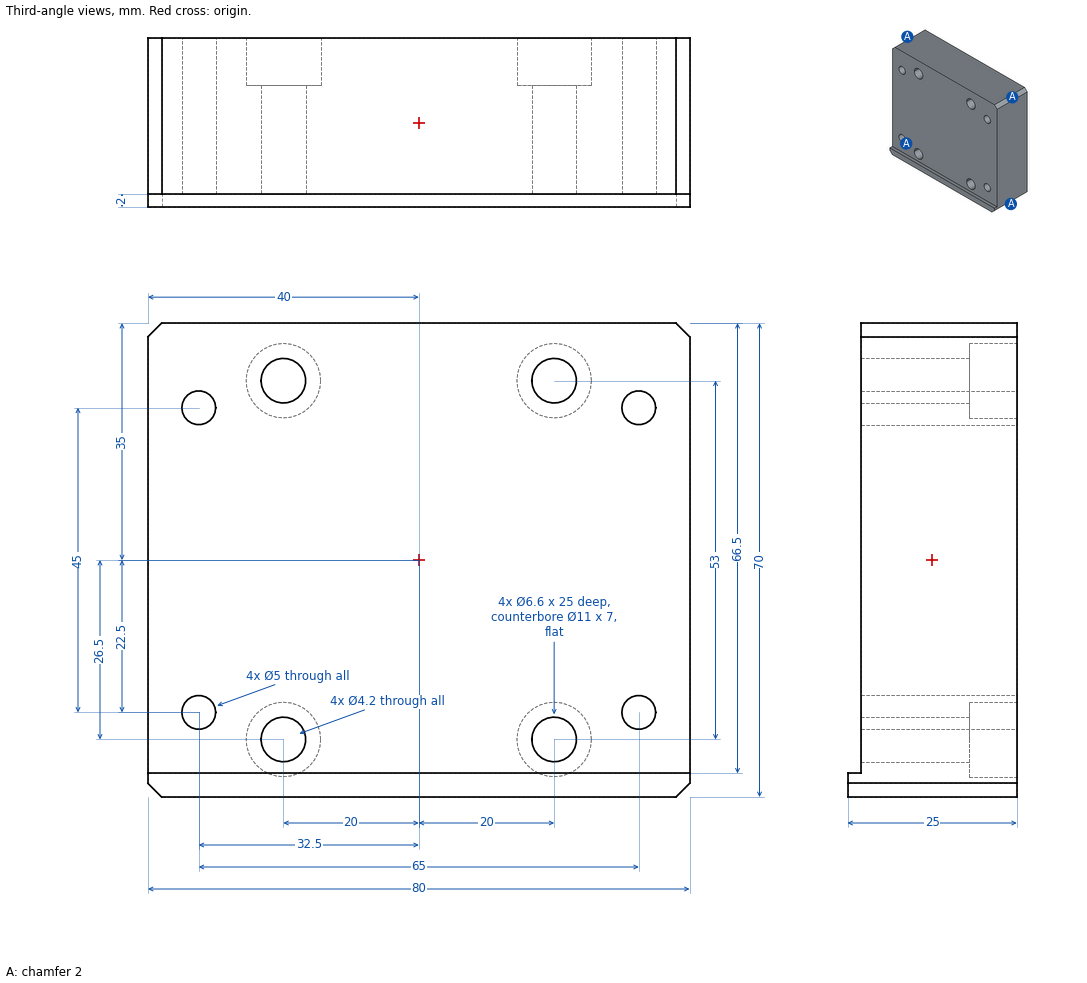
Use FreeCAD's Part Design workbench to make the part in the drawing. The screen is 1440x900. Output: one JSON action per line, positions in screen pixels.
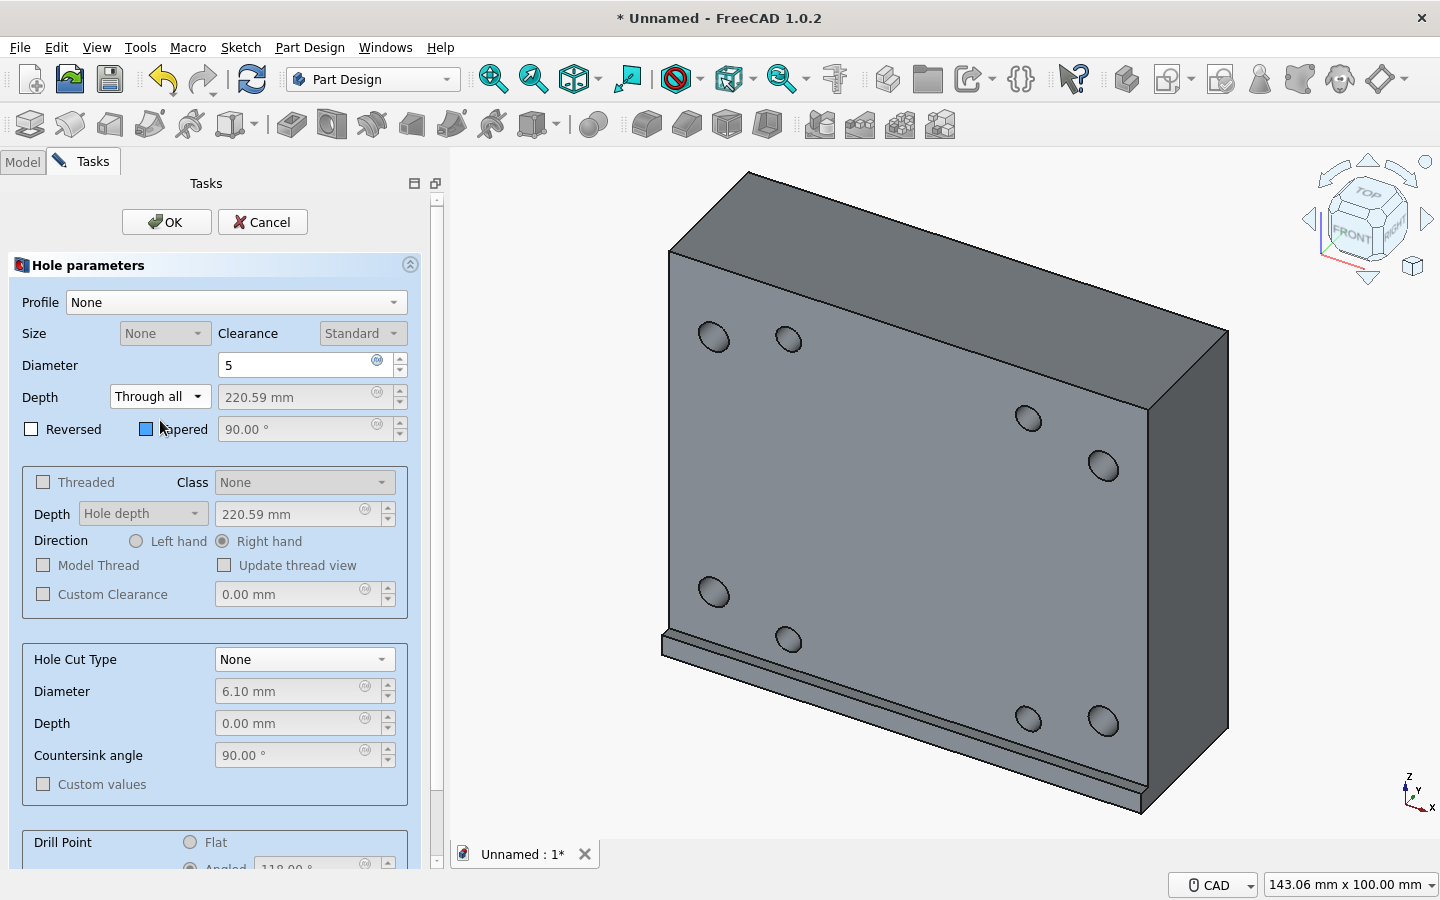
{"action": "left_click", "coordinate": [167, 222]}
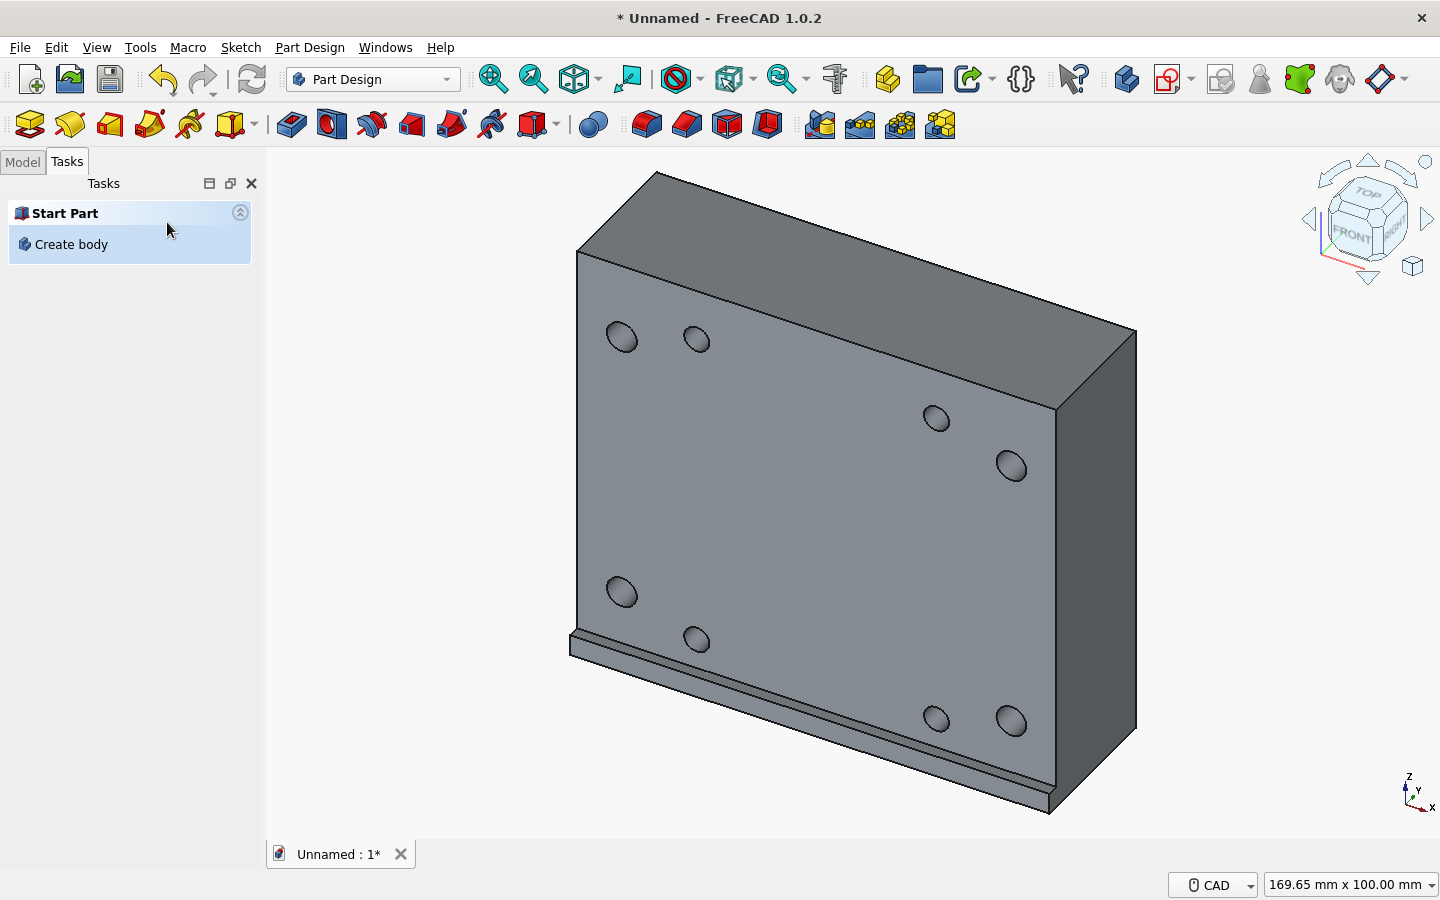
{"action": "left_click", "coordinate": [1096, 370]}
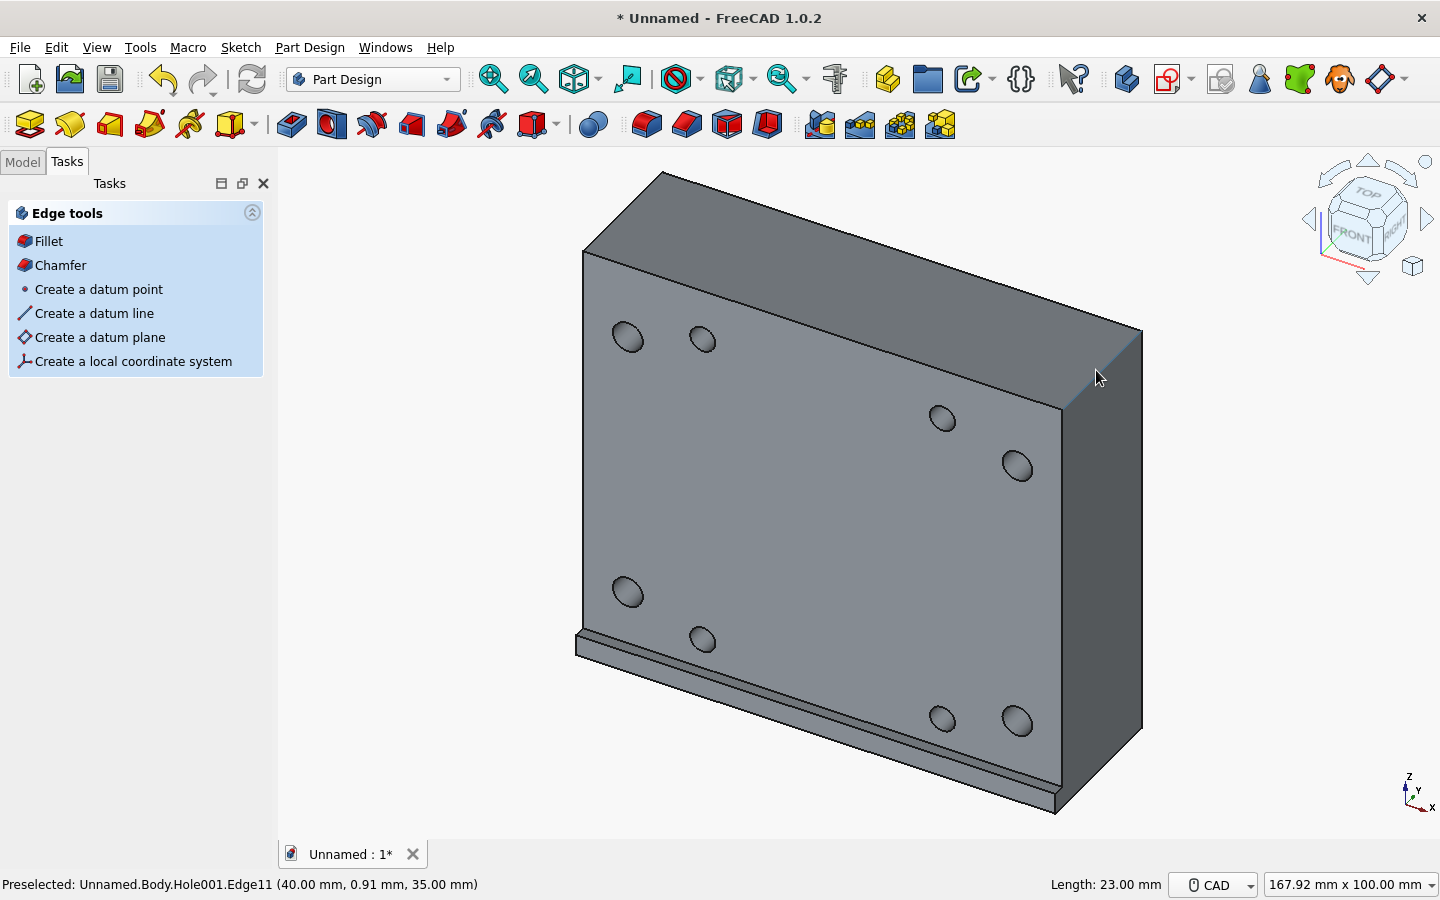
{"action": "key", "text": "0"}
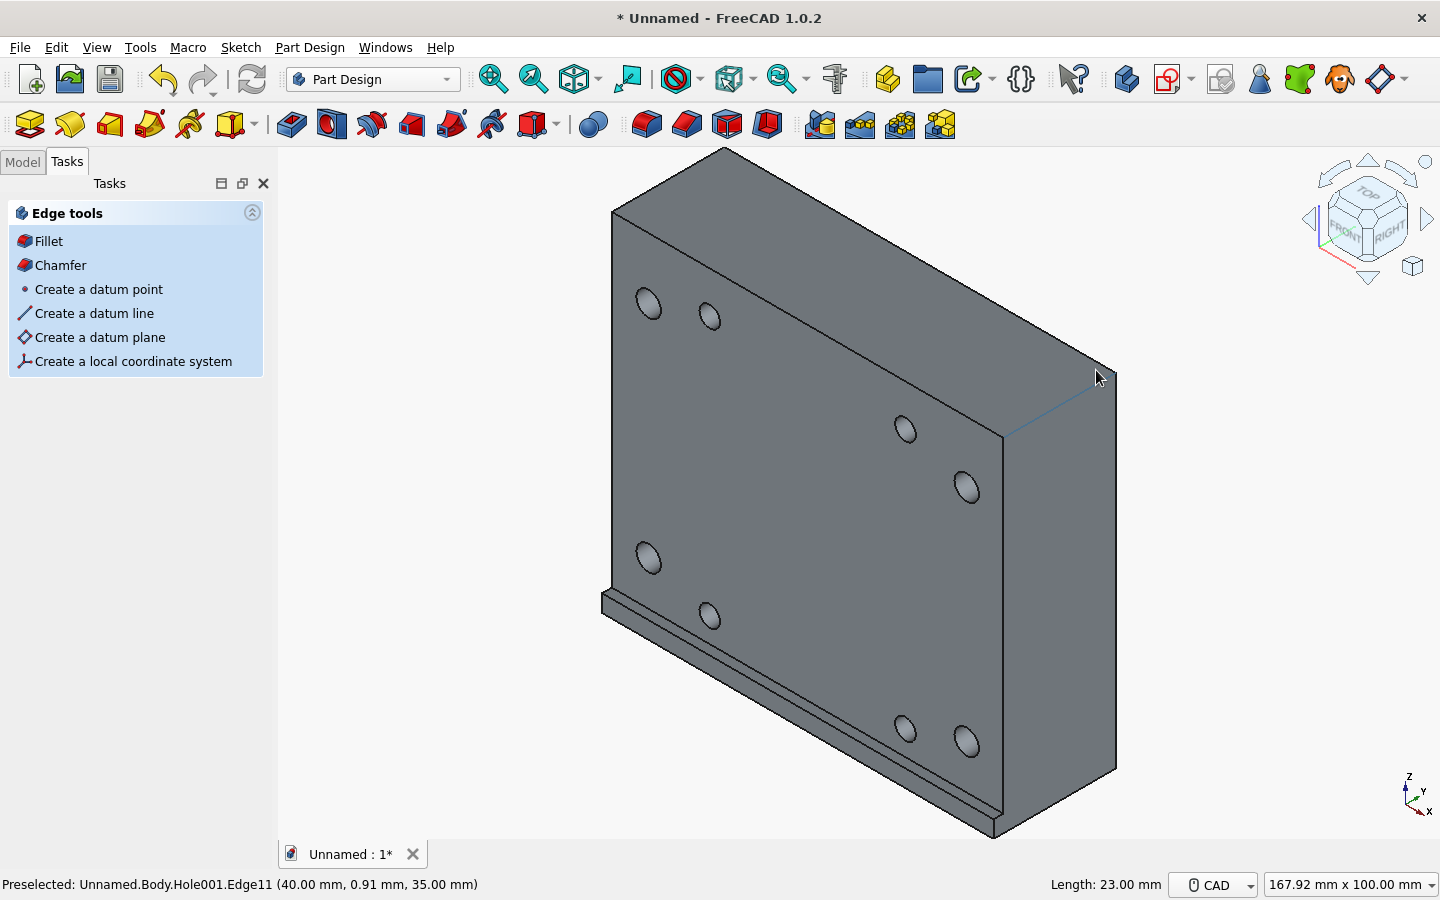
{"action": "left_click", "coordinate": [494, 80]}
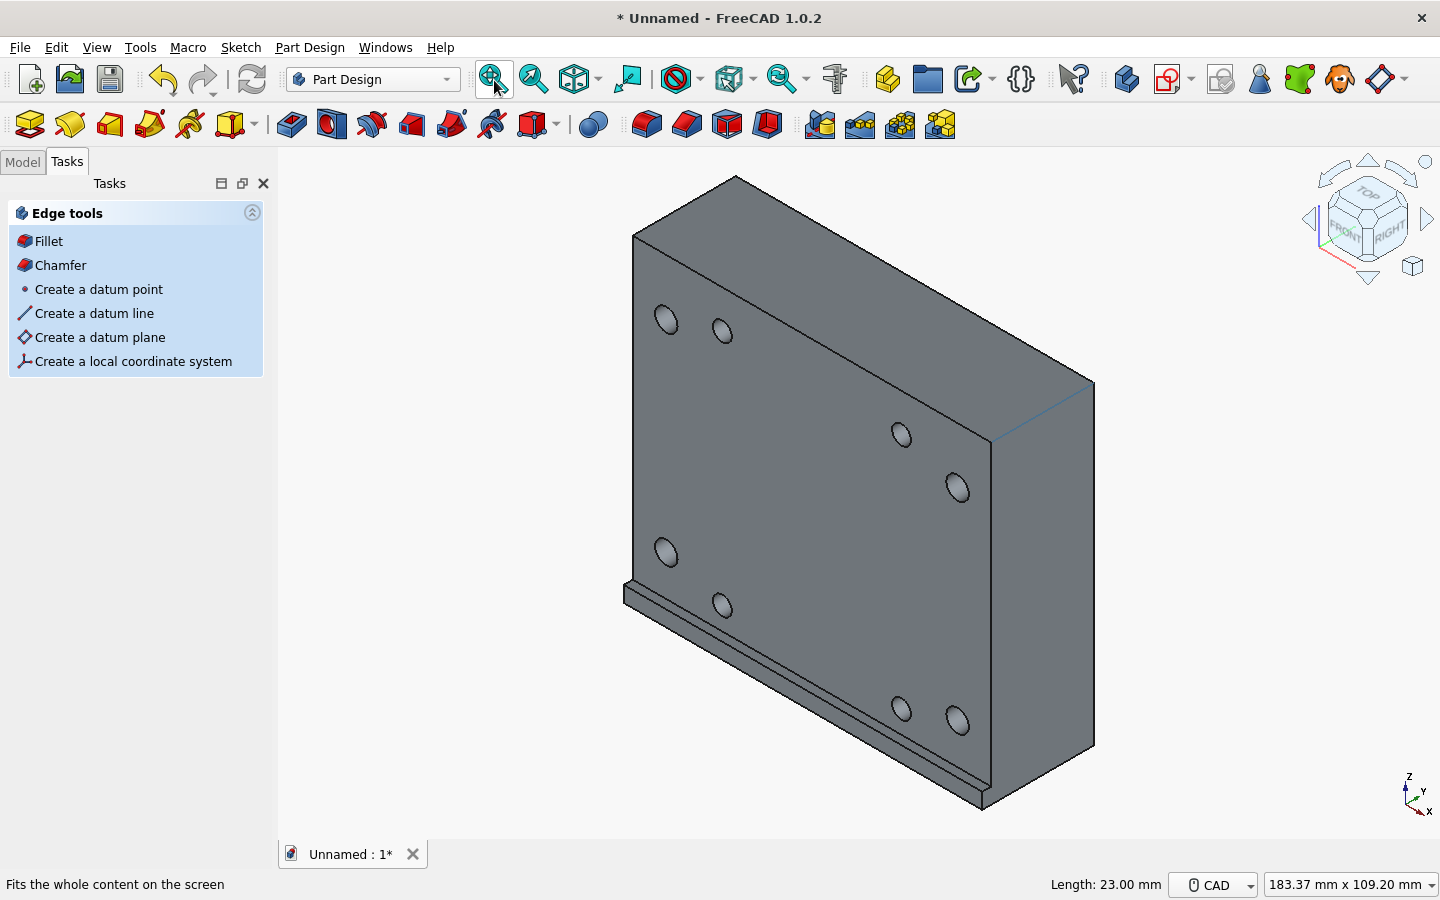
{"action": "key", "text": "2"}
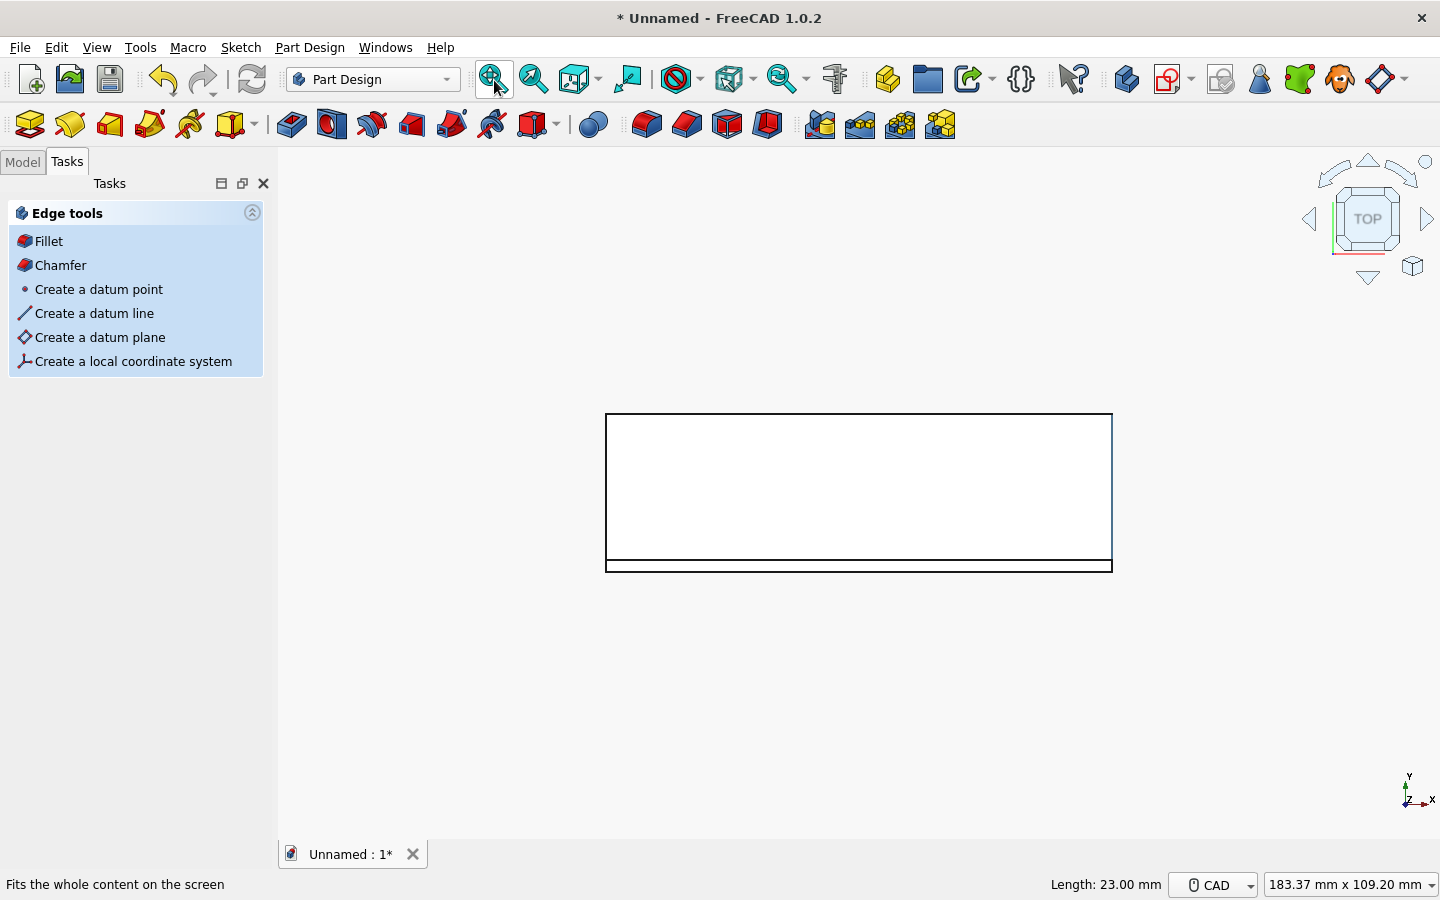
{"action": "left_click", "coordinate": [494, 80]}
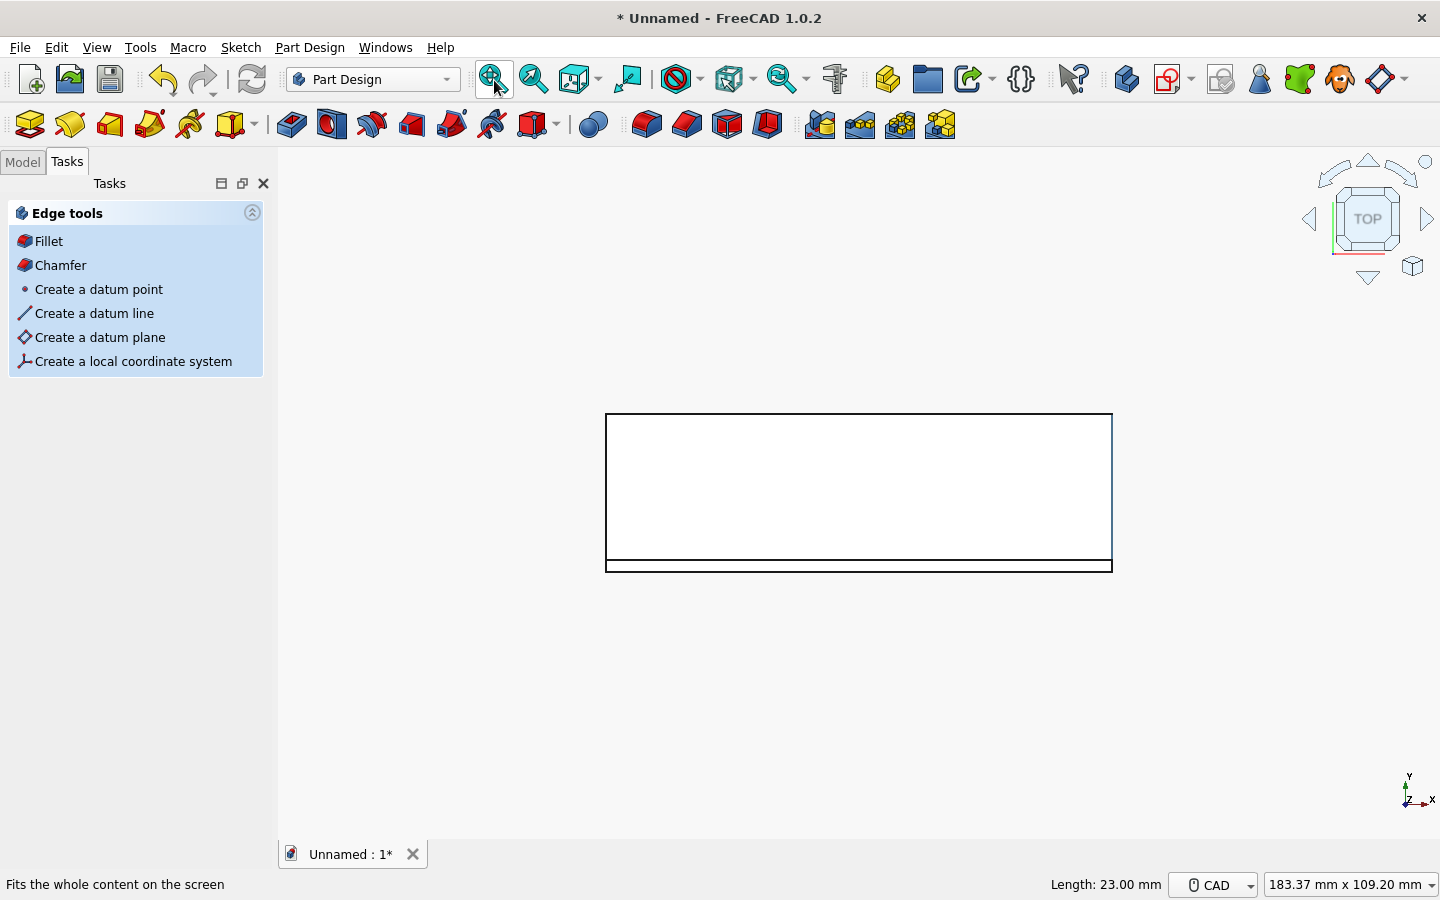
{"action": "left_click", "coordinate": [606, 486], "text": "ctrl"}